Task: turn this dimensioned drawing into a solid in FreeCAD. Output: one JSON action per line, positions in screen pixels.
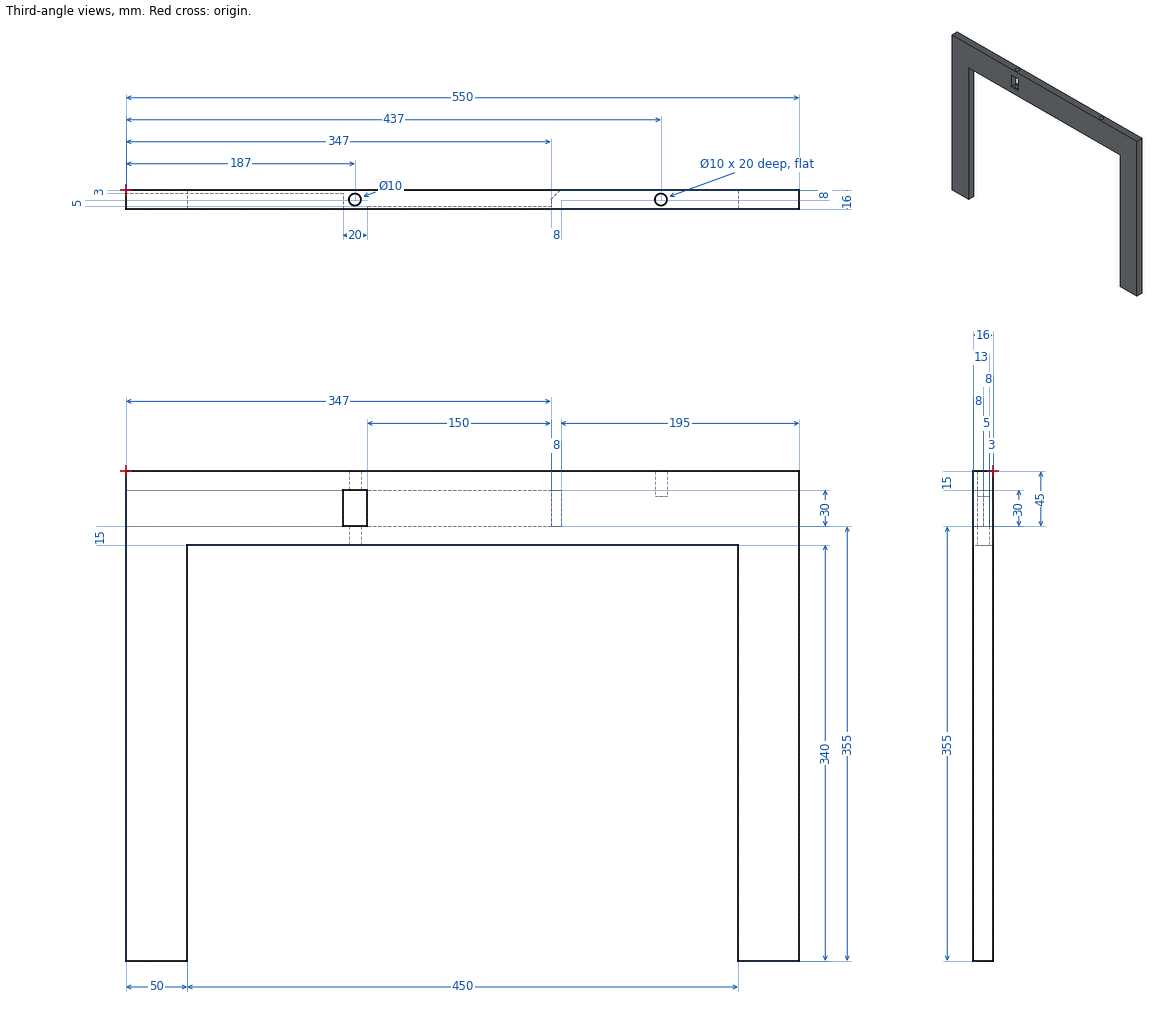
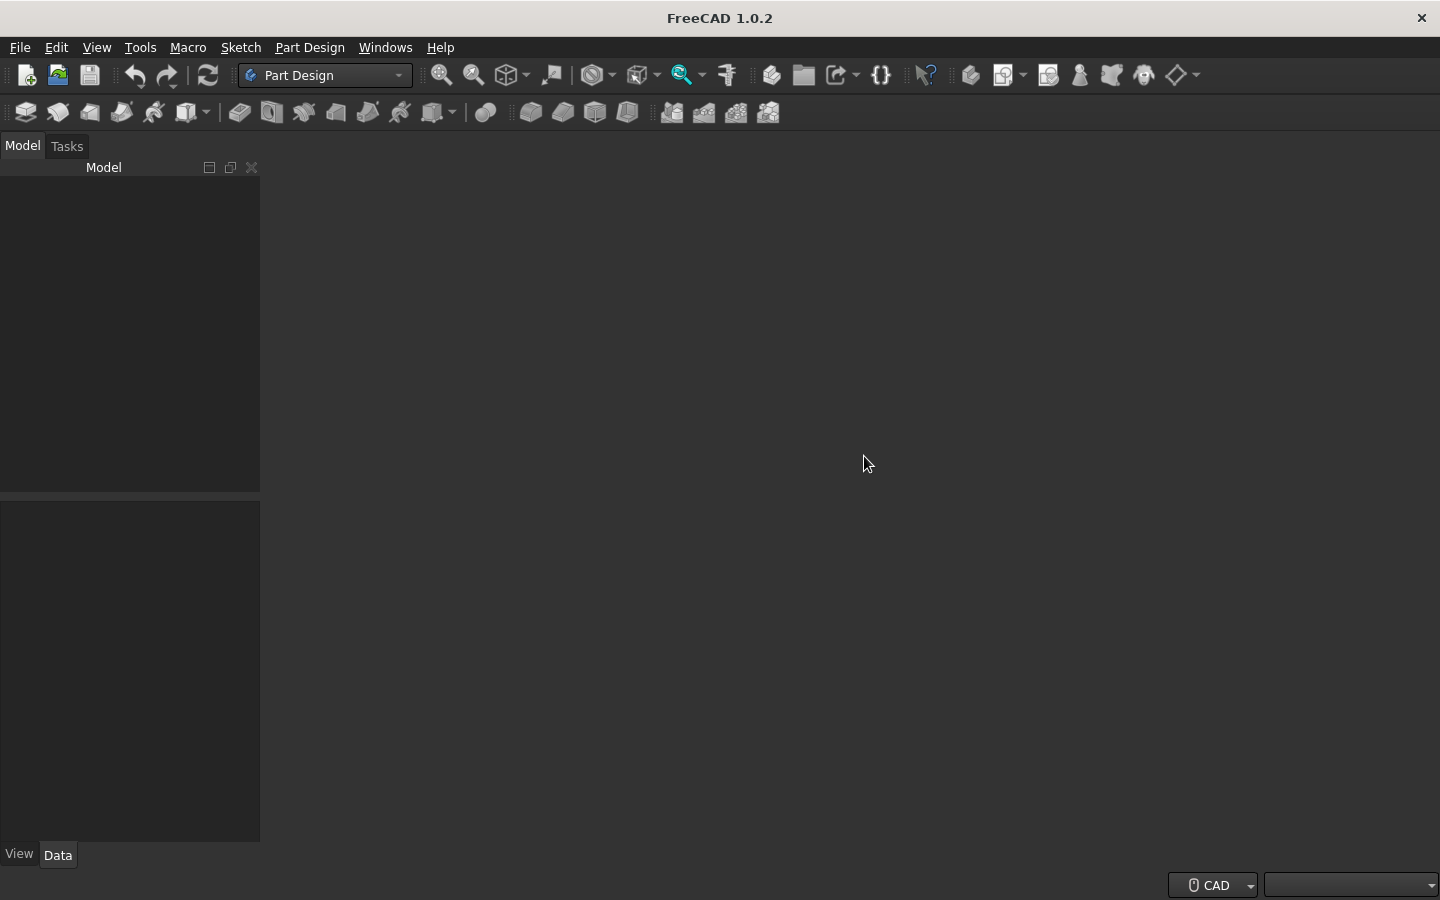
{"action": "left_click", "coordinate": [26, 76]}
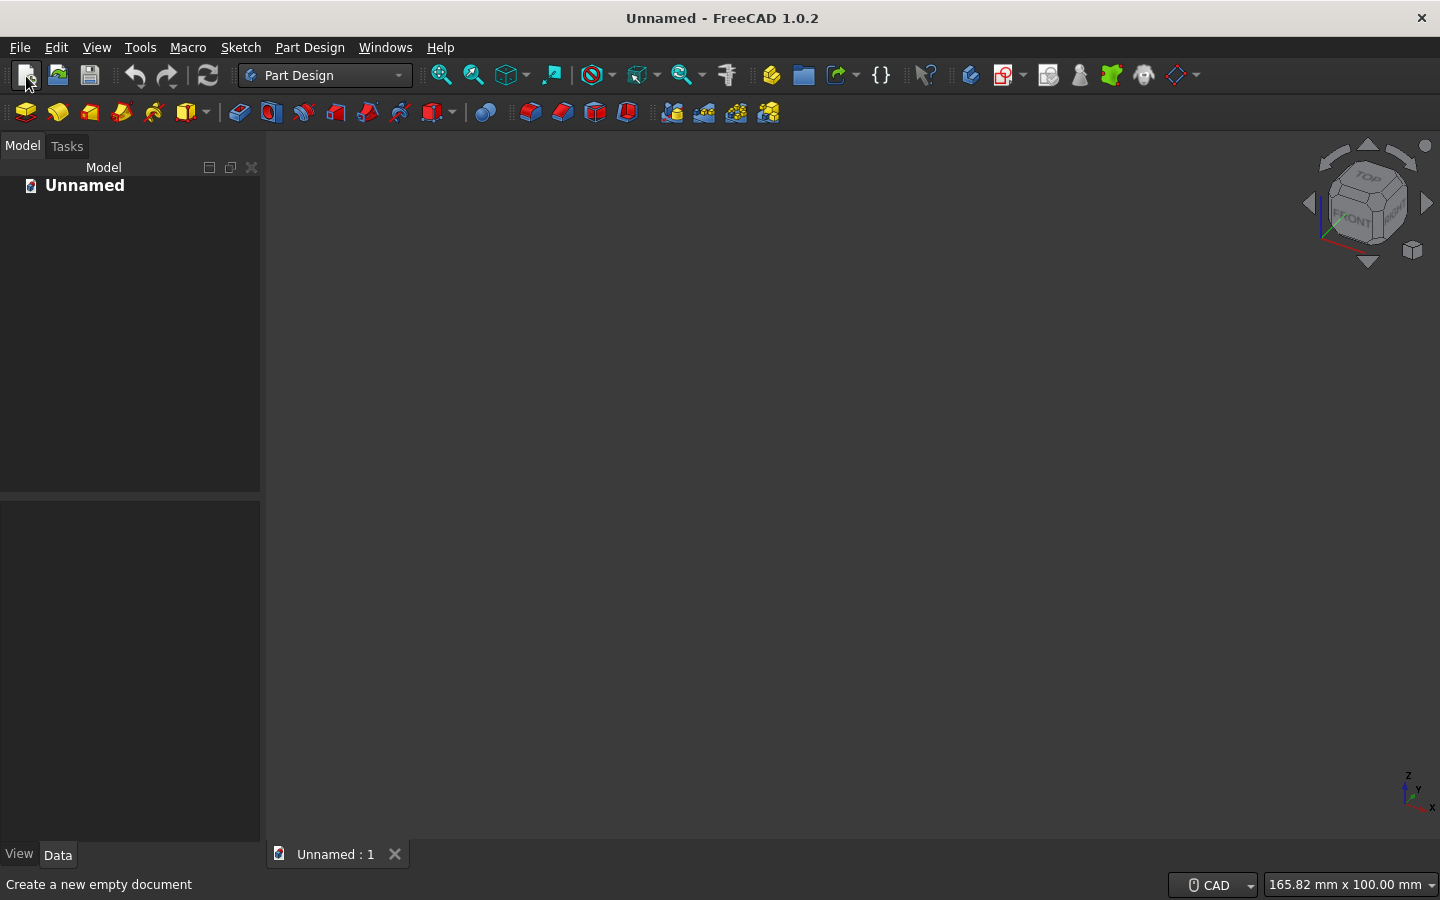
{"action": "left_click", "coordinate": [972, 76]}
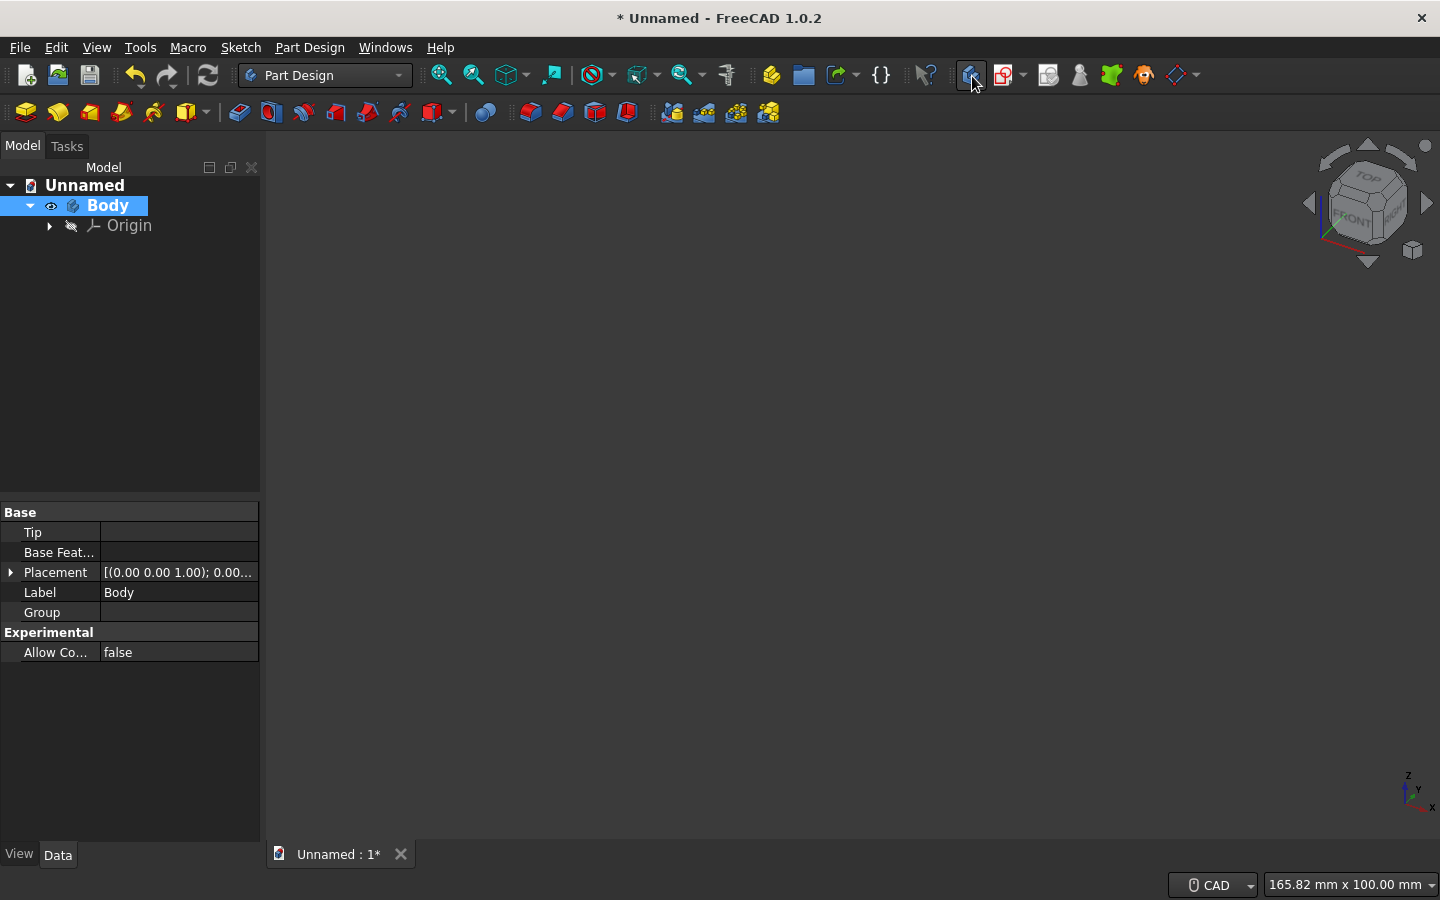
{"action": "left_click", "coordinate": [50, 226]}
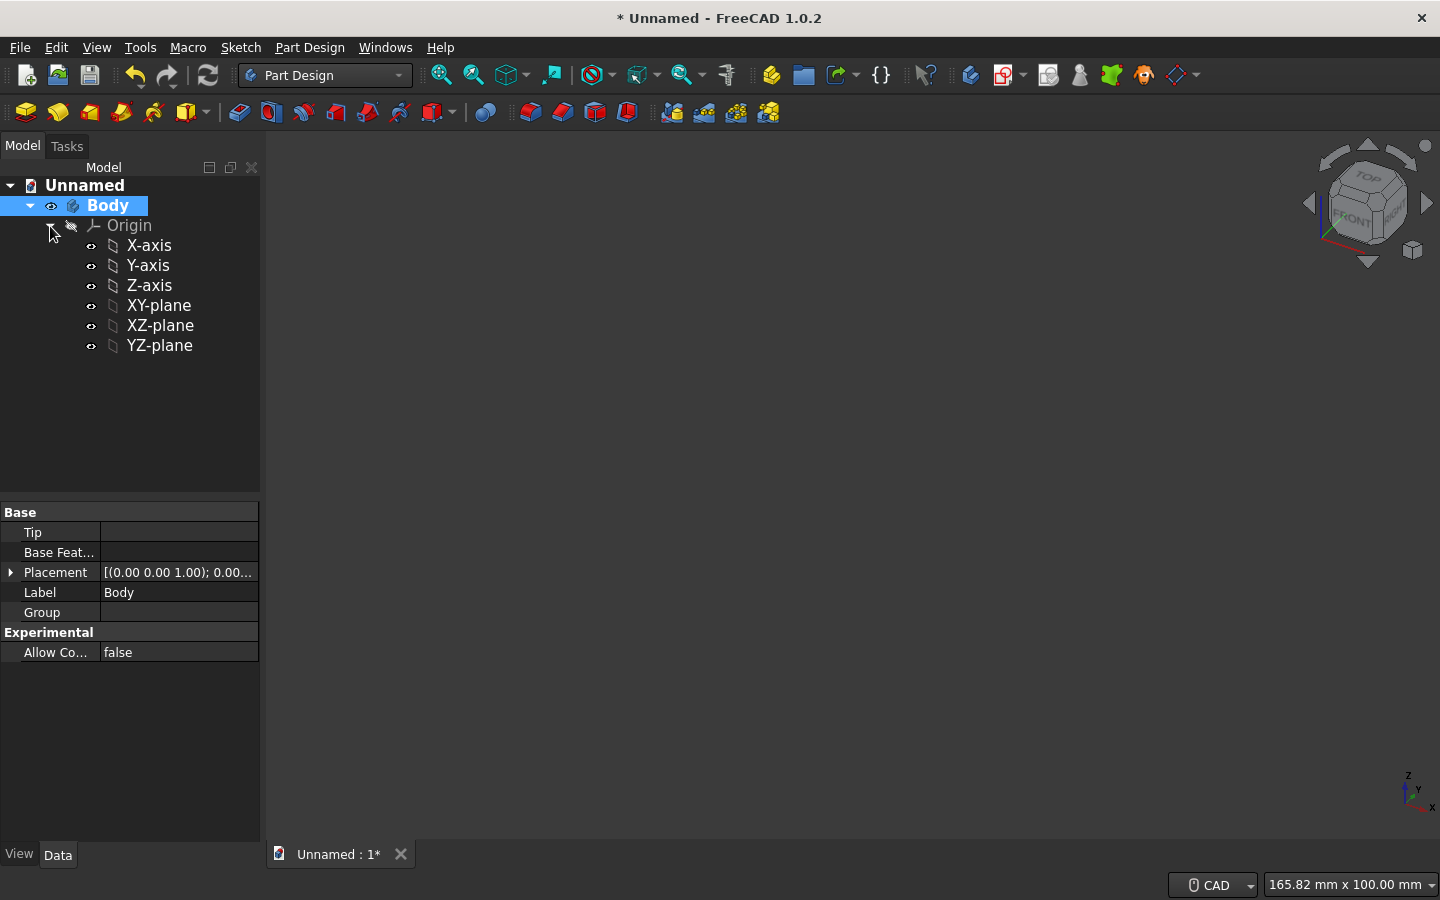
{"action": "left_click", "coordinate": [136, 306]}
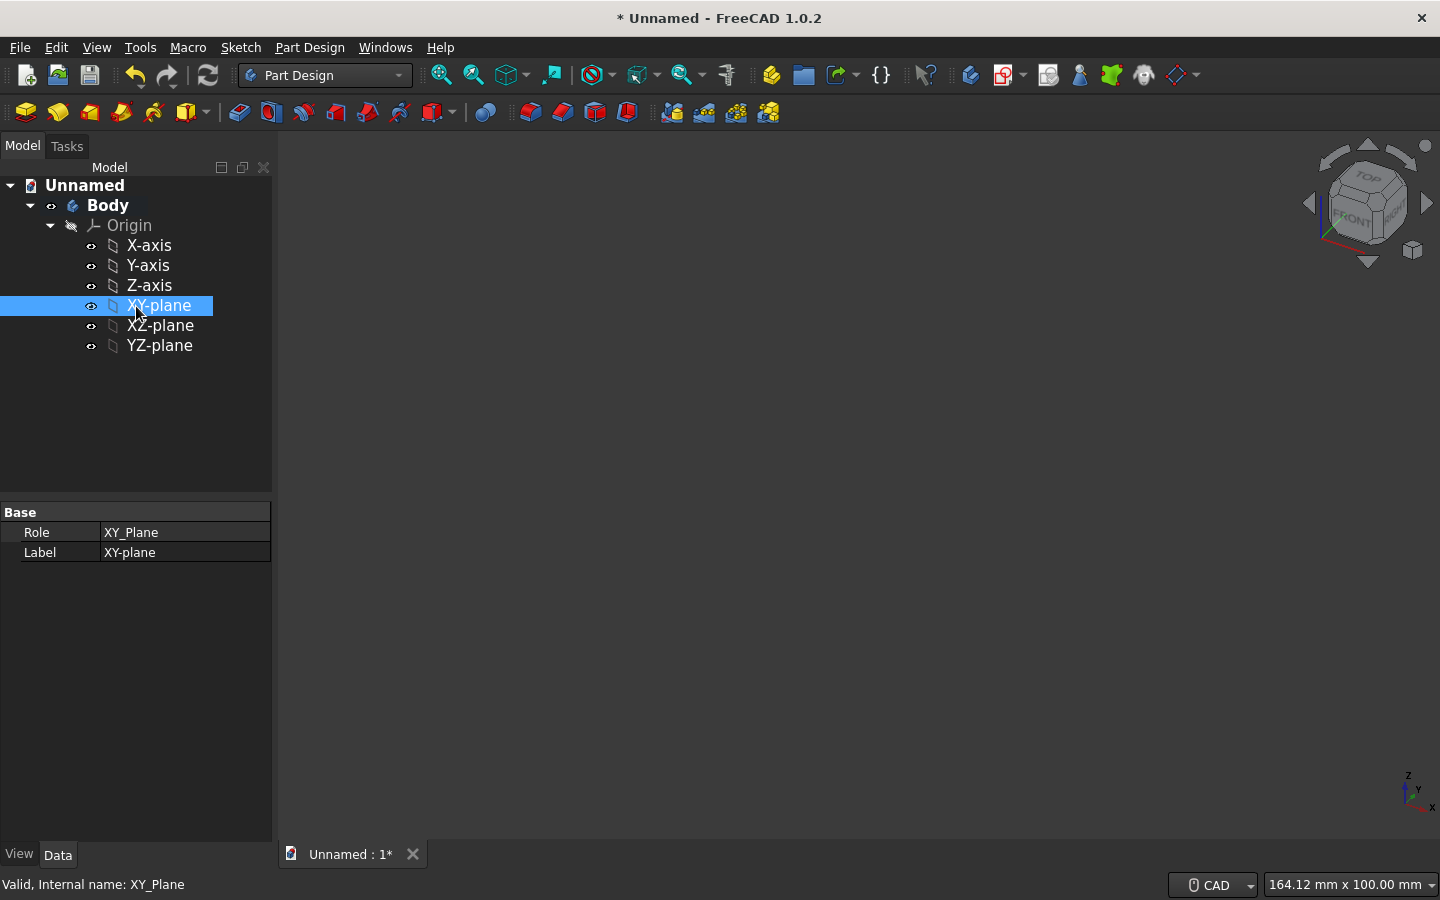
{"action": "left_click", "coordinate": [1176, 76]}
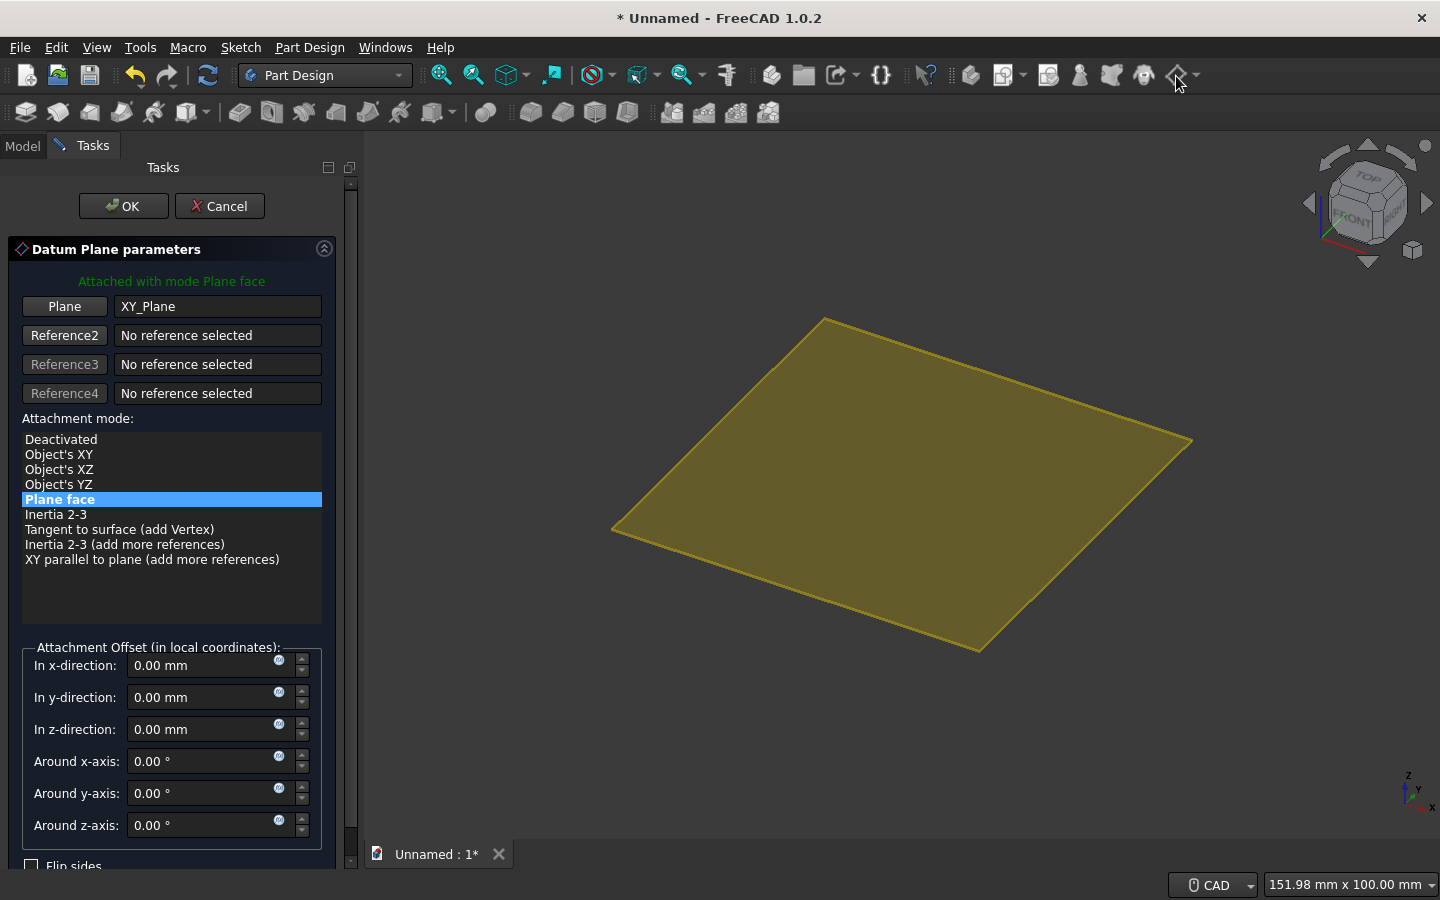
{"action": "triple_click", "coordinate": [210, 729]}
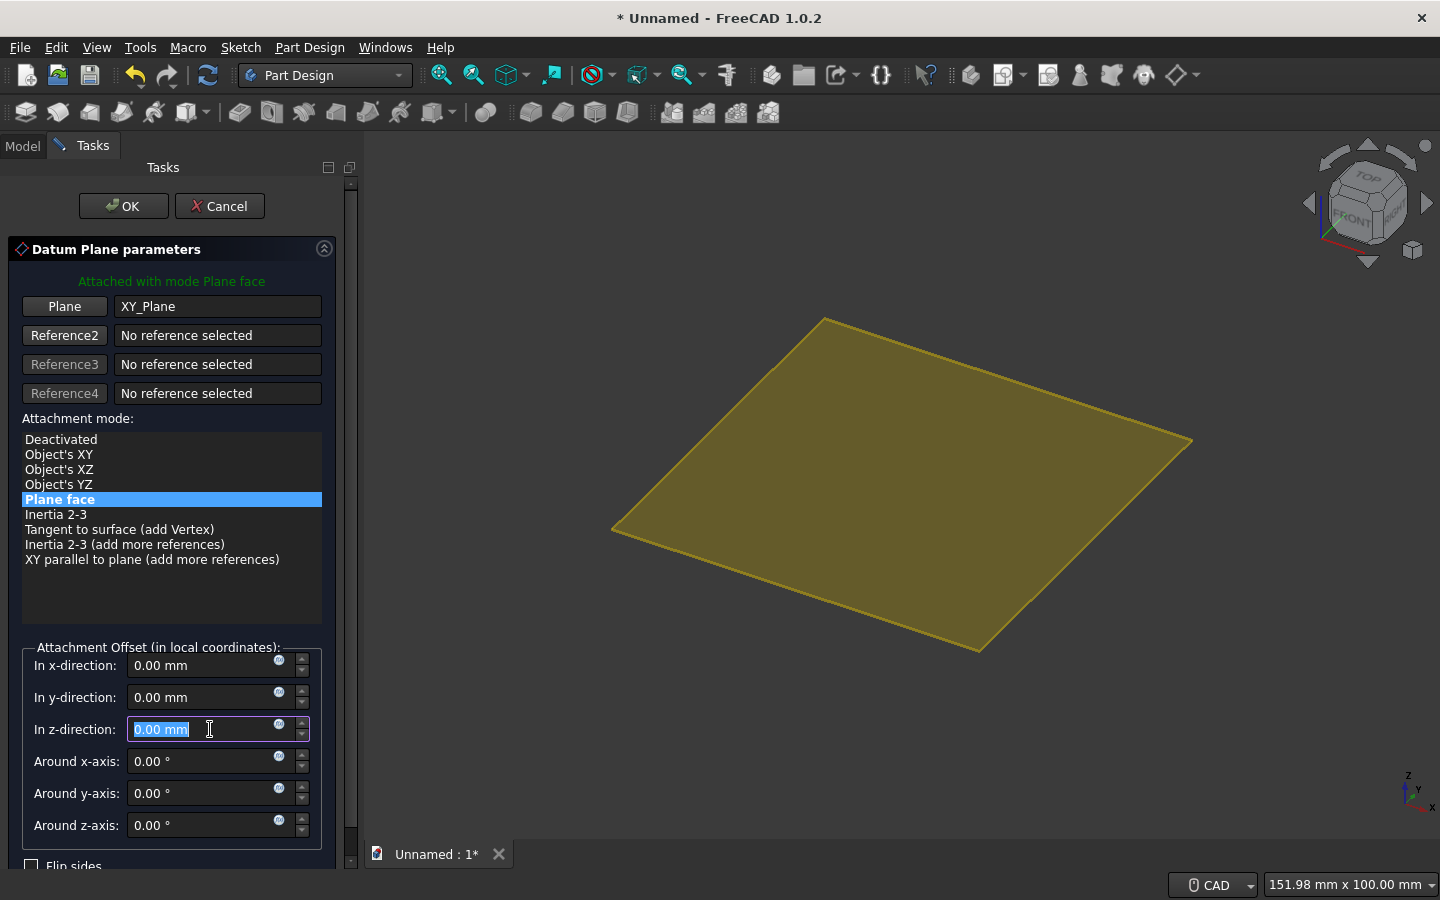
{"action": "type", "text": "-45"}
{"action": "key", "text": "Tab"}